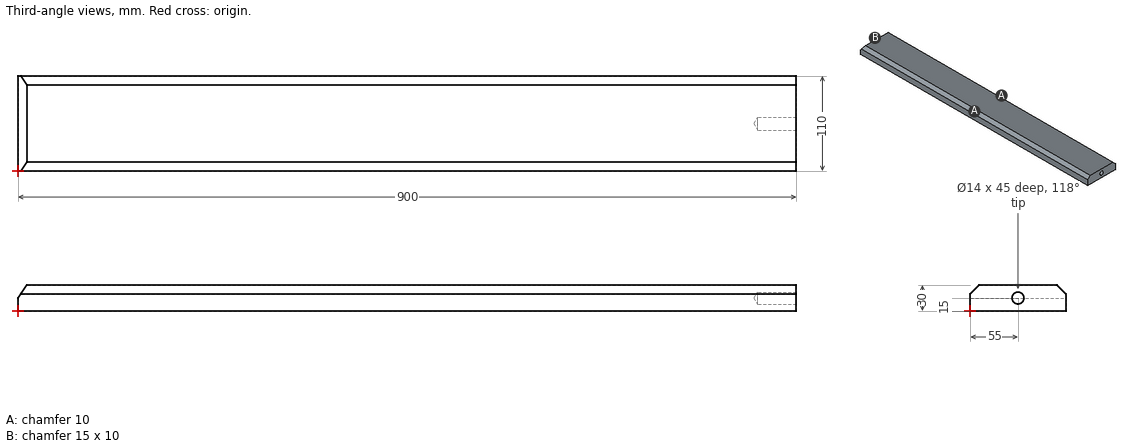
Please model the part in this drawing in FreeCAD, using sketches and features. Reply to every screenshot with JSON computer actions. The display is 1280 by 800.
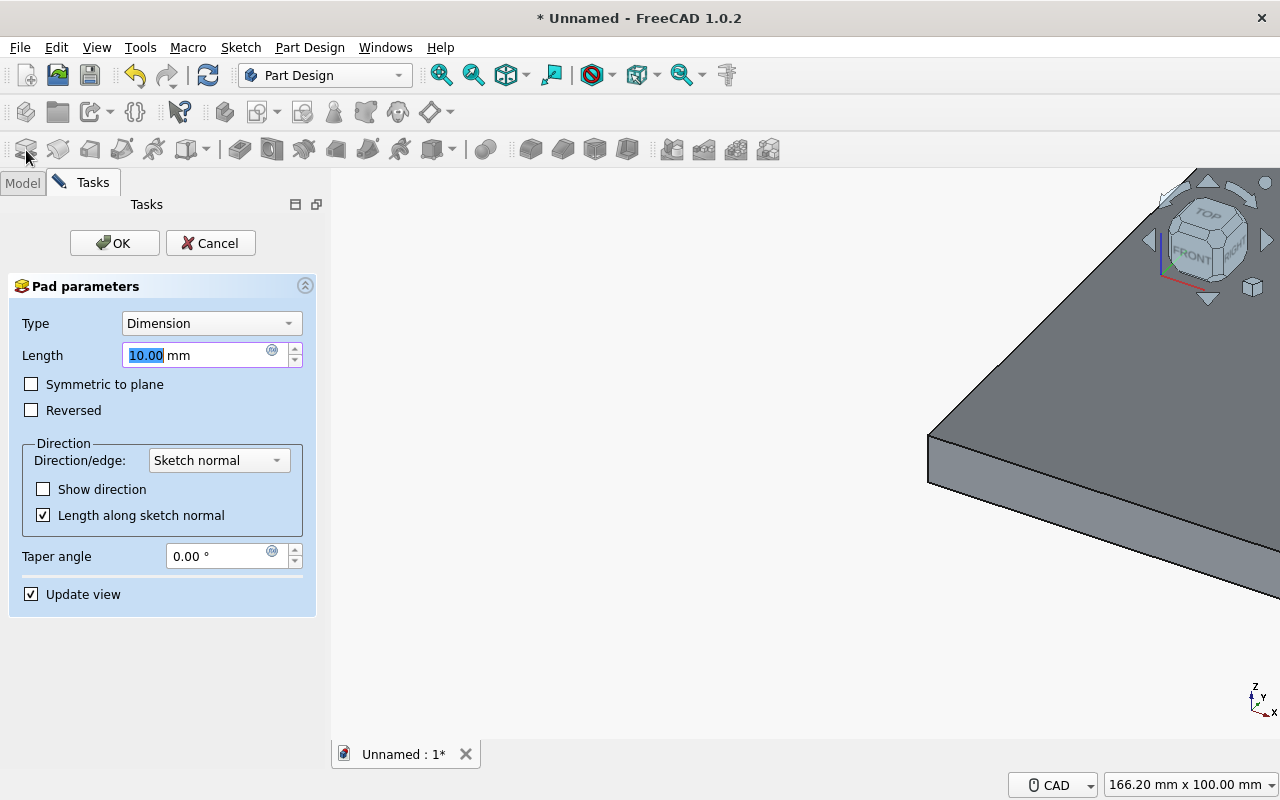
{"action": "type", "text": "30"}
{"action": "key", "text": "Tab"}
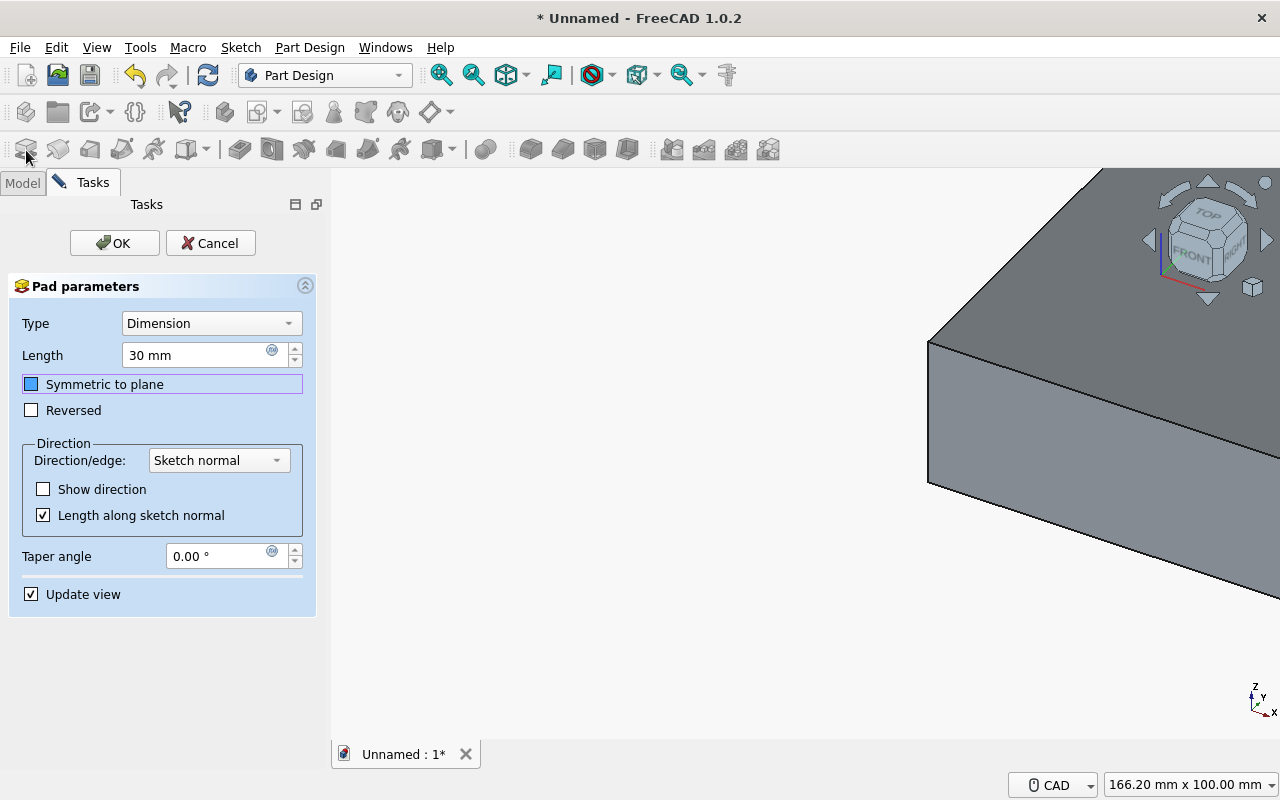
{"action": "left_click", "coordinate": [115, 243]}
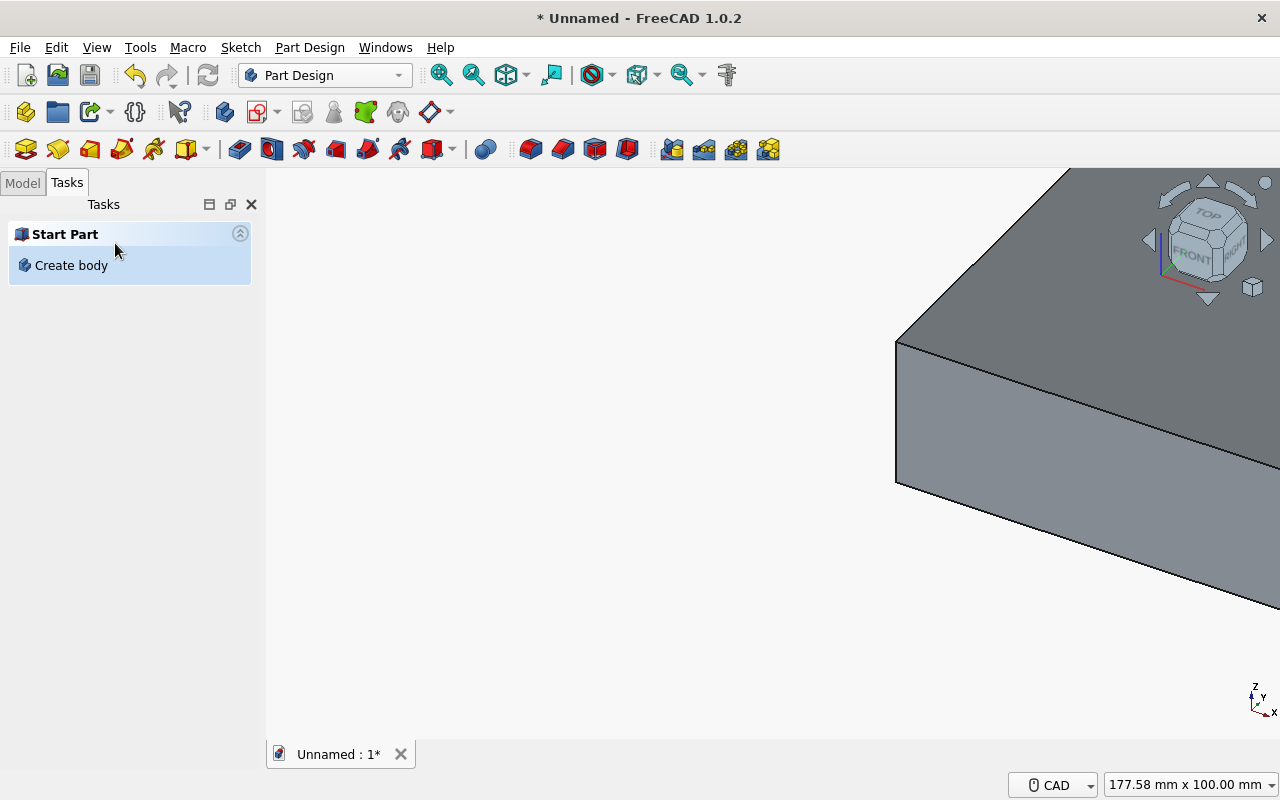
{"action": "key", "text": "v f"}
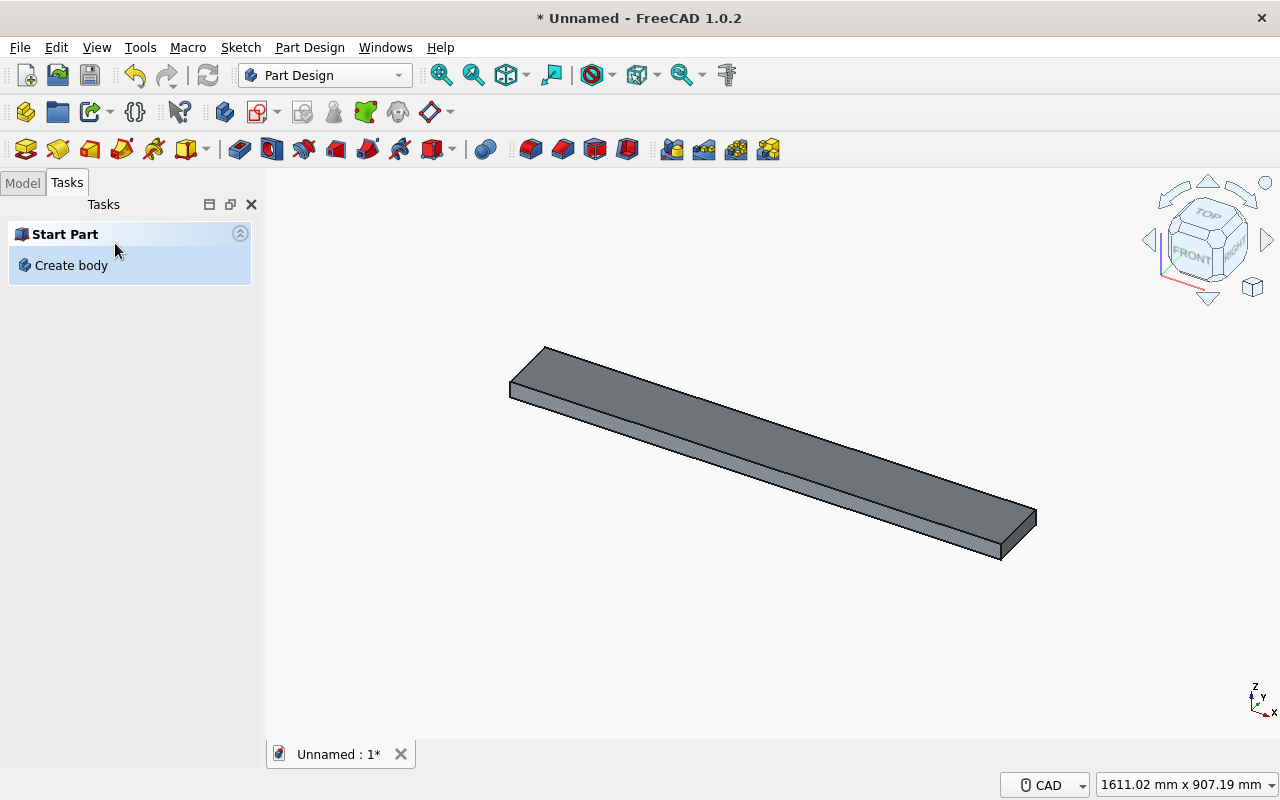
{"action": "left_click", "coordinate": [756, 462]}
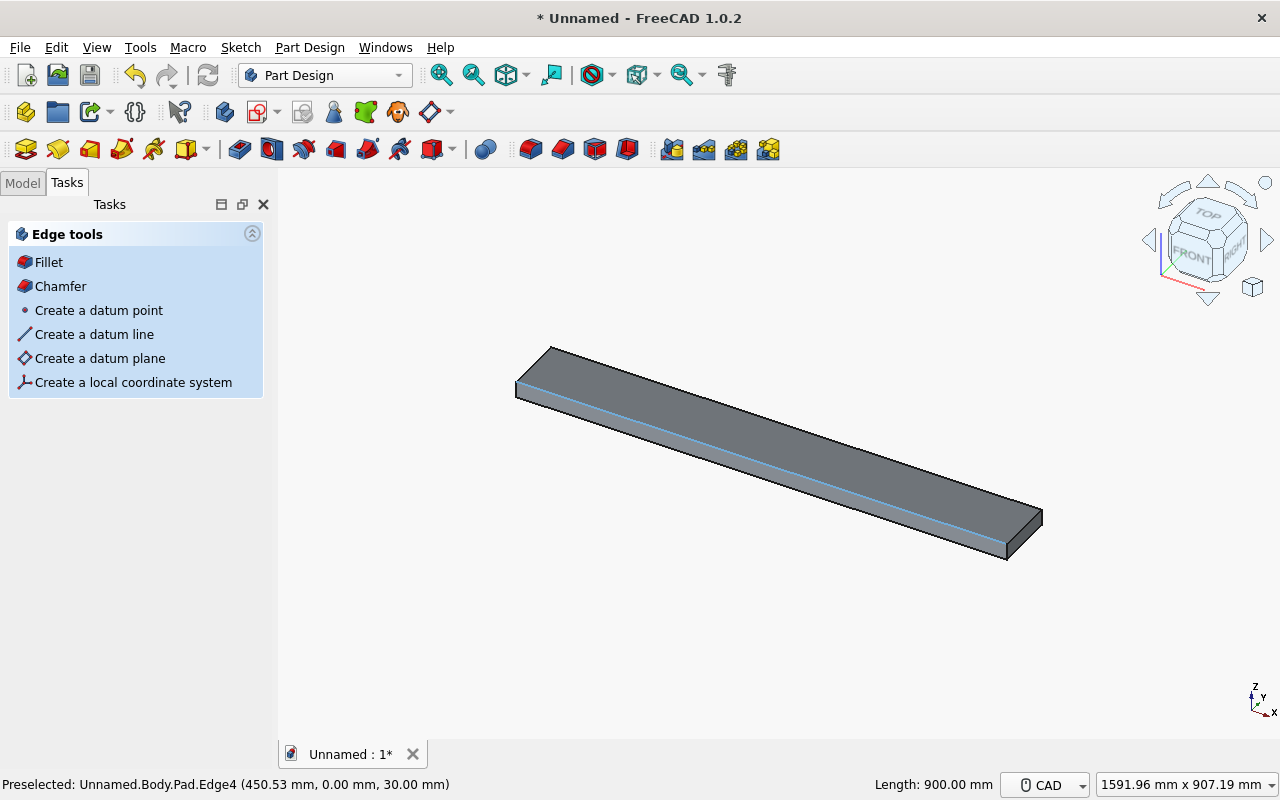
{"action": "key", "text": "0"}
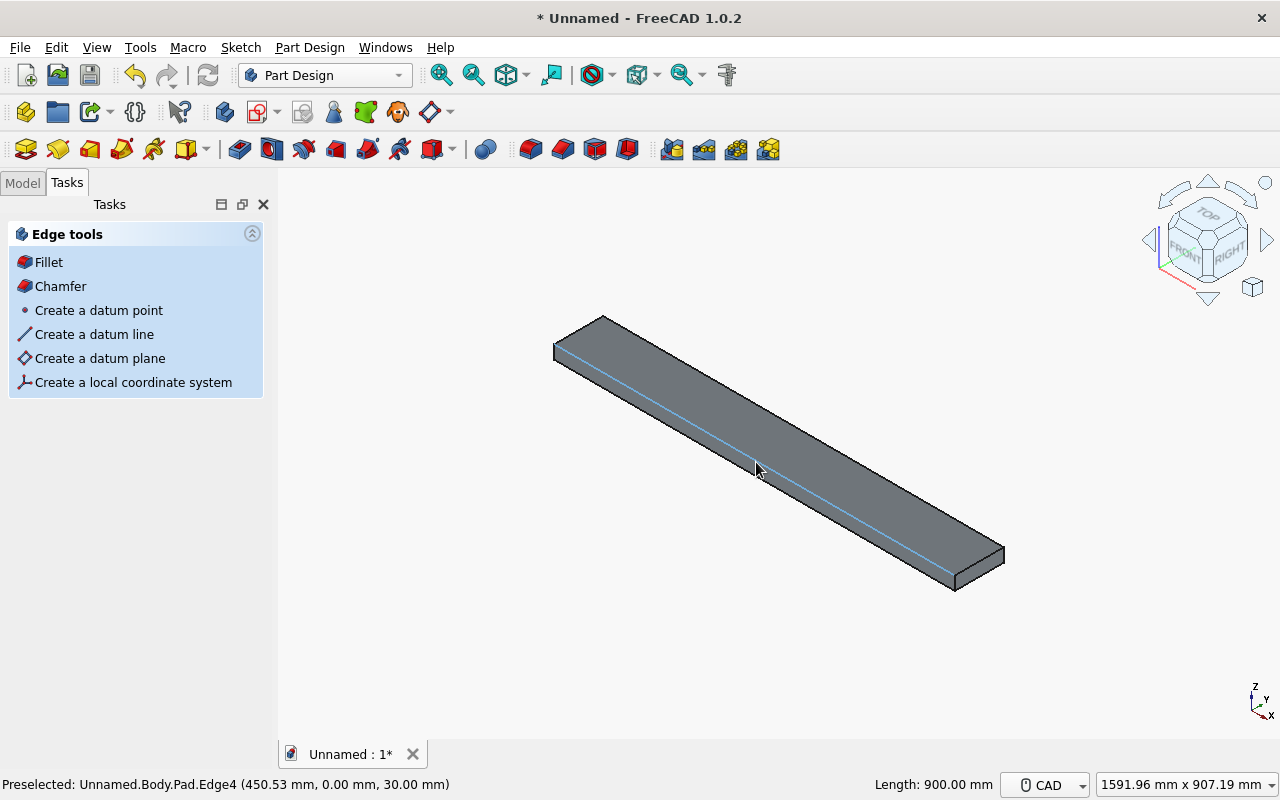
{"action": "key", "text": "2"}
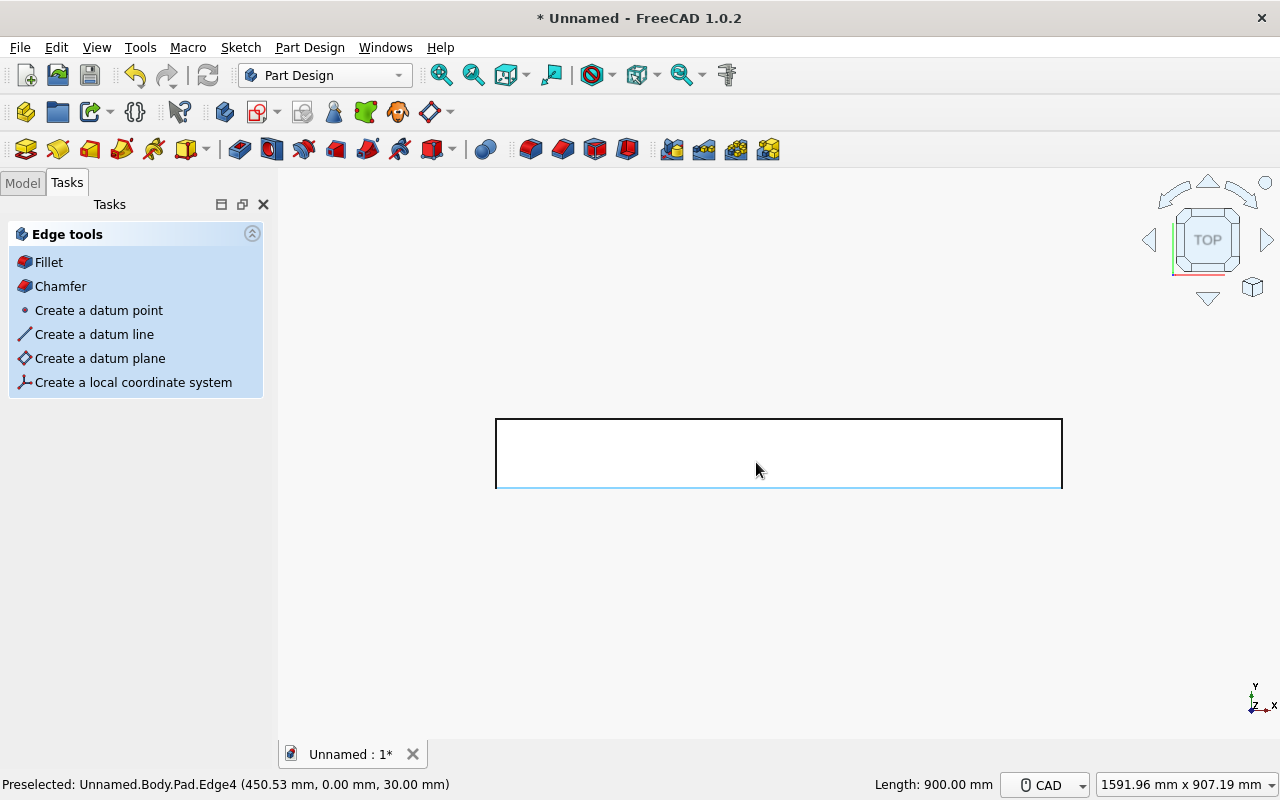
{"action": "left_click", "coordinate": [779, 418], "text": "ctrl"}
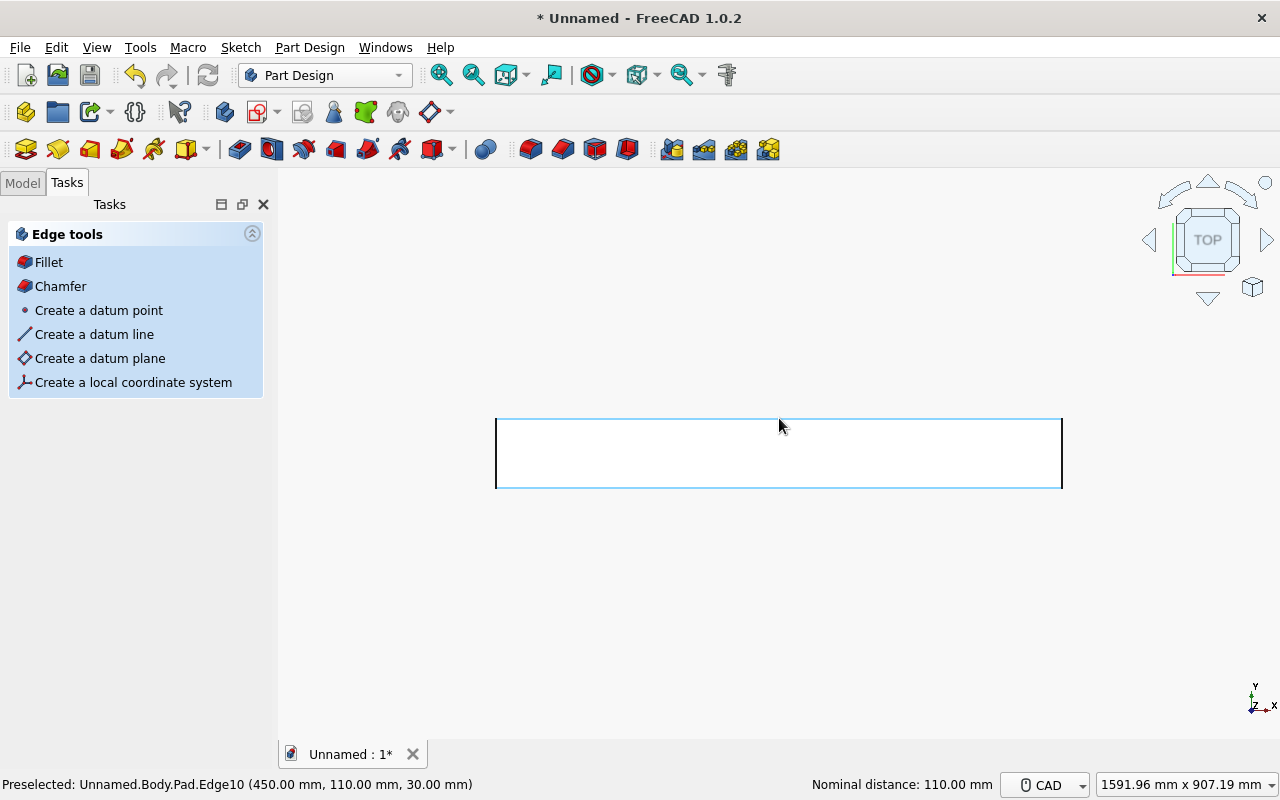
{"action": "left_click", "coordinate": [564, 150]}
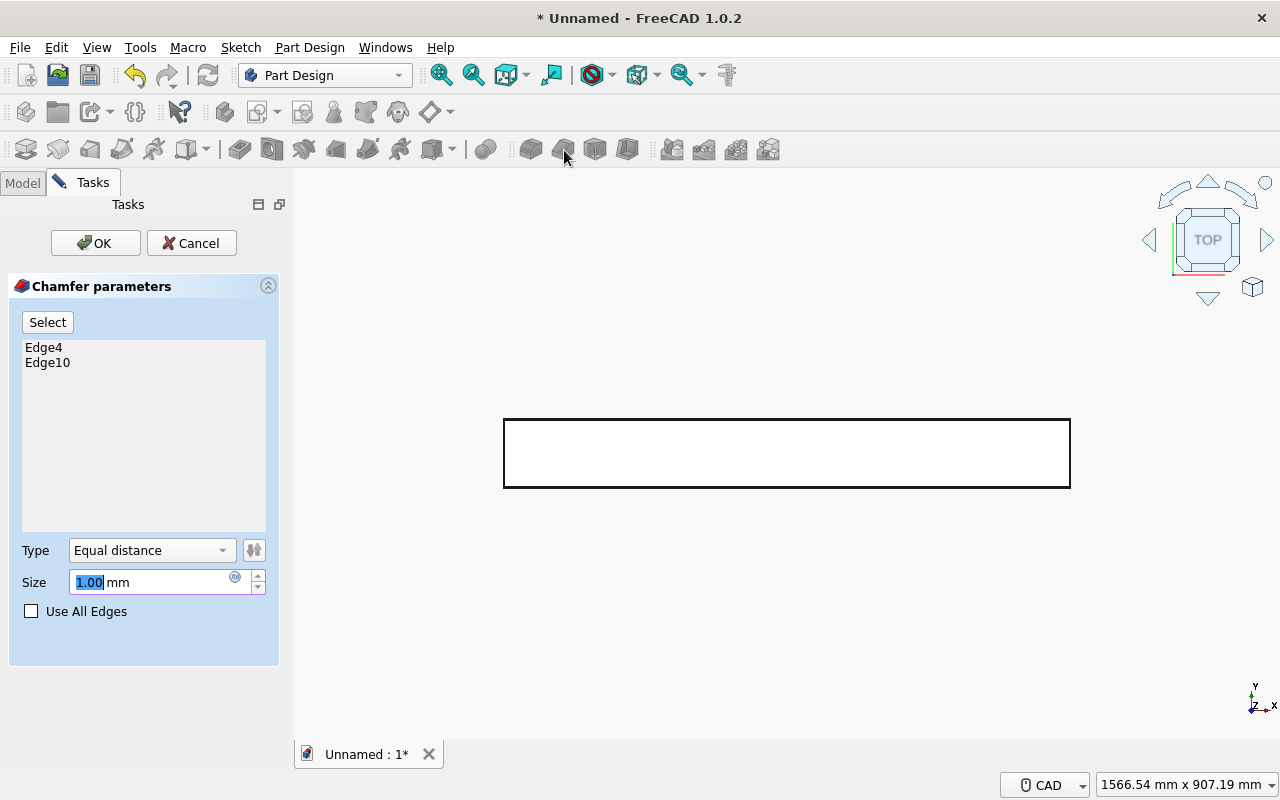
{"action": "type", "text": "10"}
{"action": "key", "text": "Tab"}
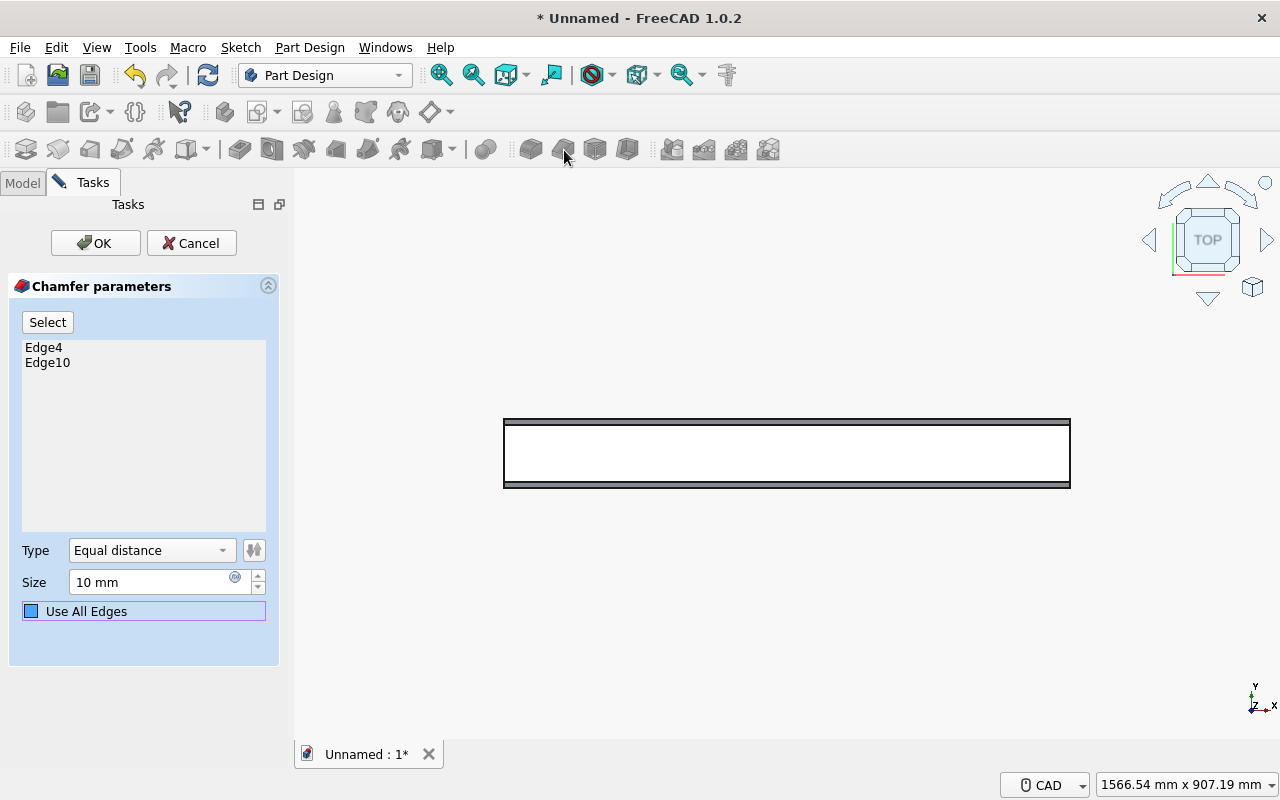
{"action": "left_click", "coordinate": [96, 243]}